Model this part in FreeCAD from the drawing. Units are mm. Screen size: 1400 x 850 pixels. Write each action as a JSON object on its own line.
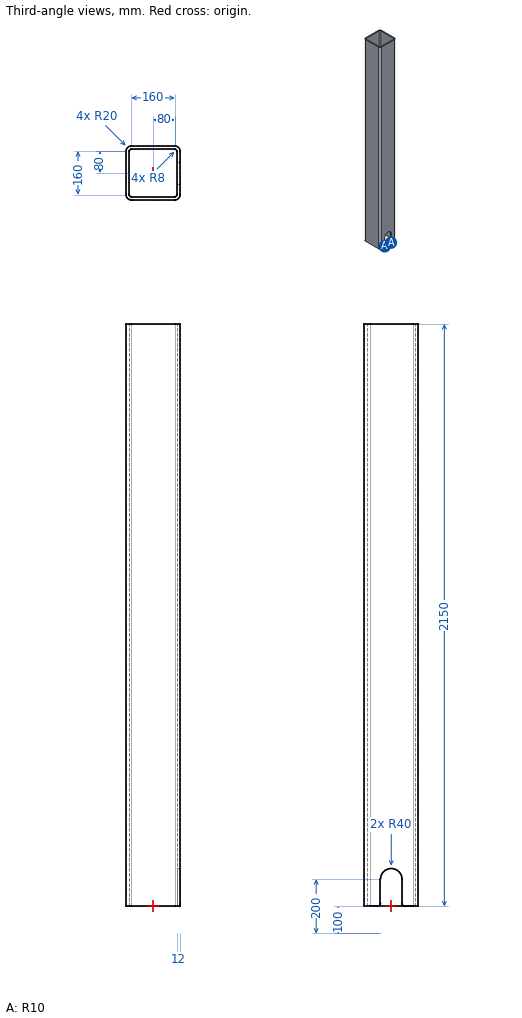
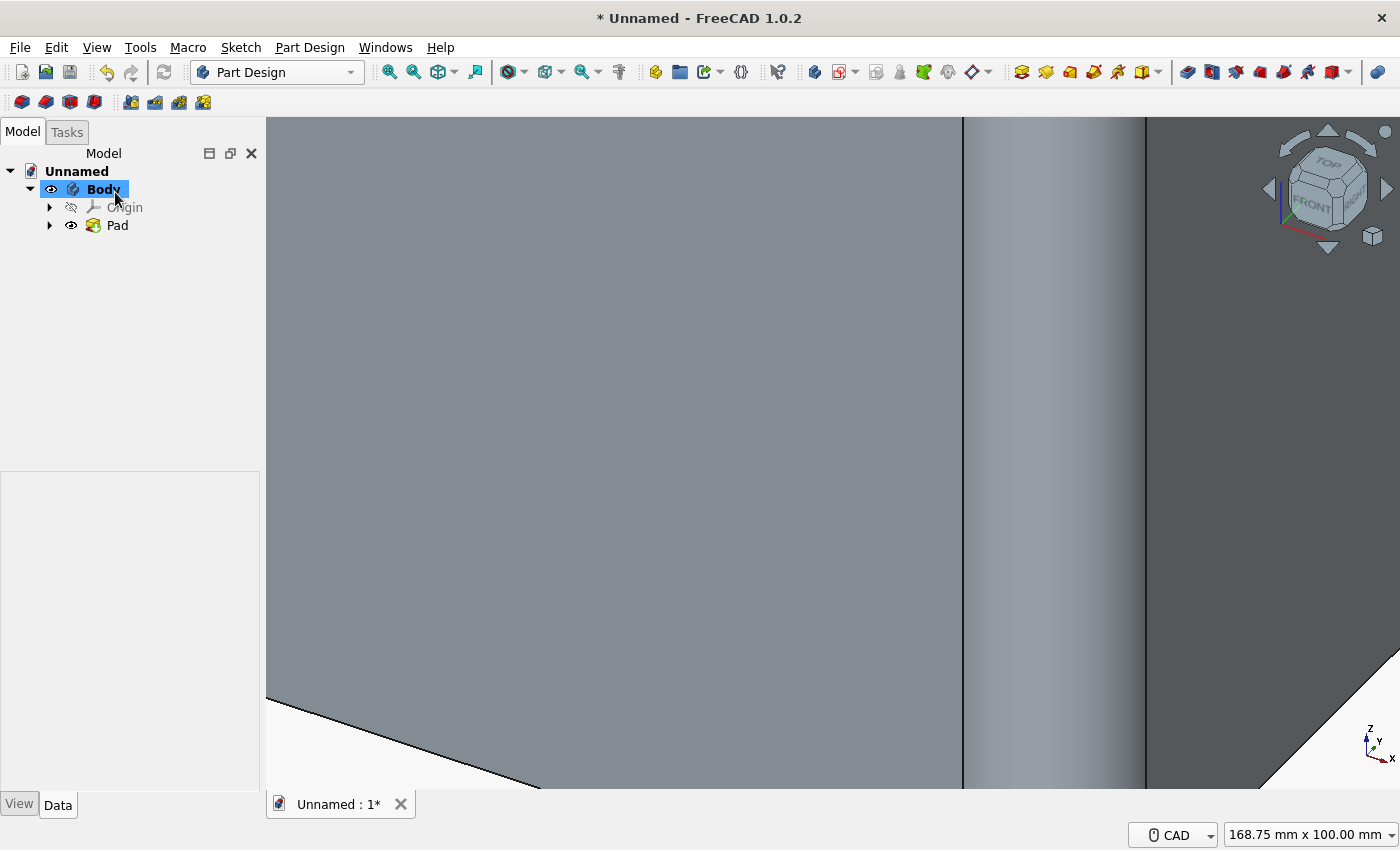
{"action": "left_click", "coordinate": [390, 72]}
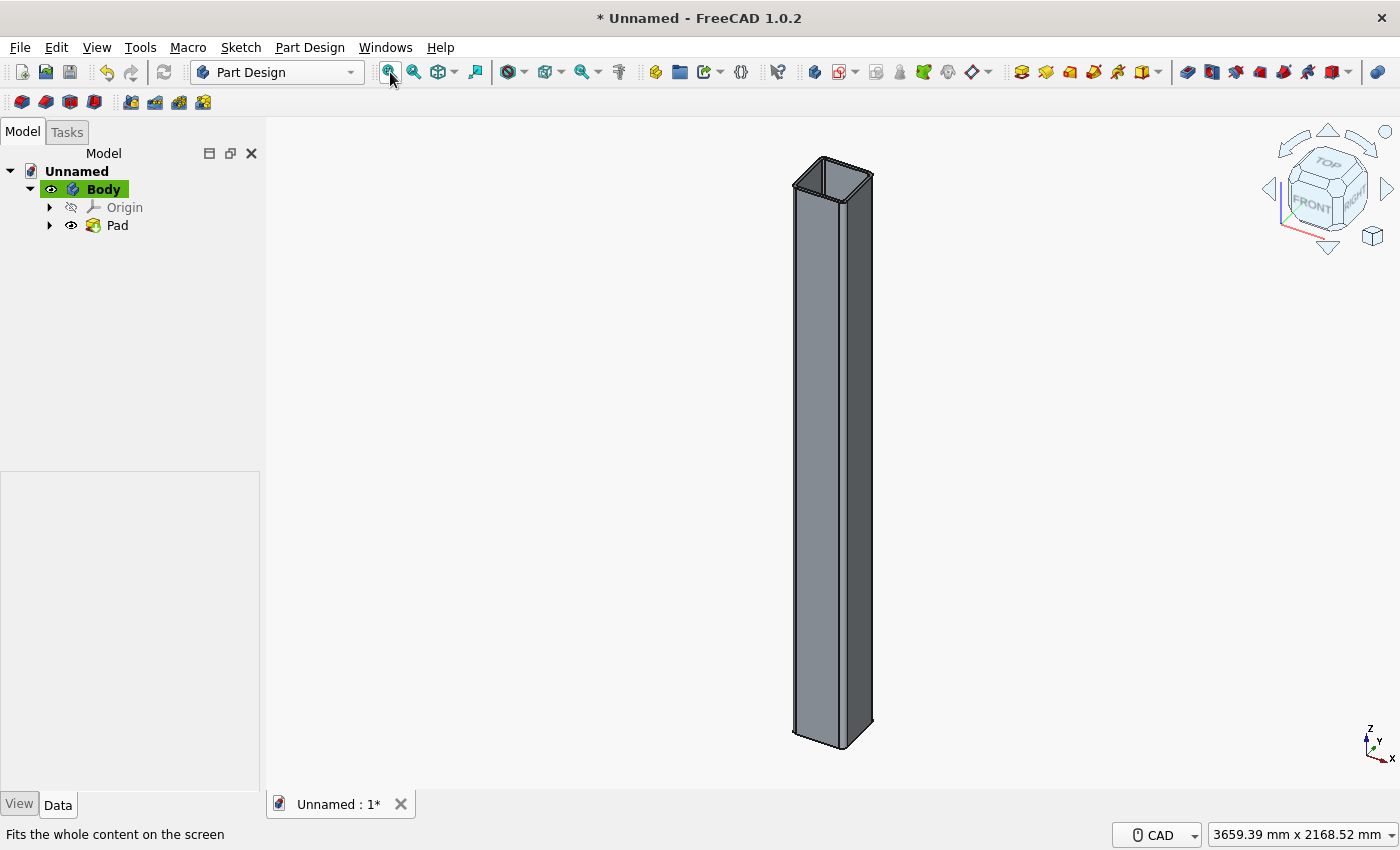
{"action": "left_click", "coordinate": [860, 227]}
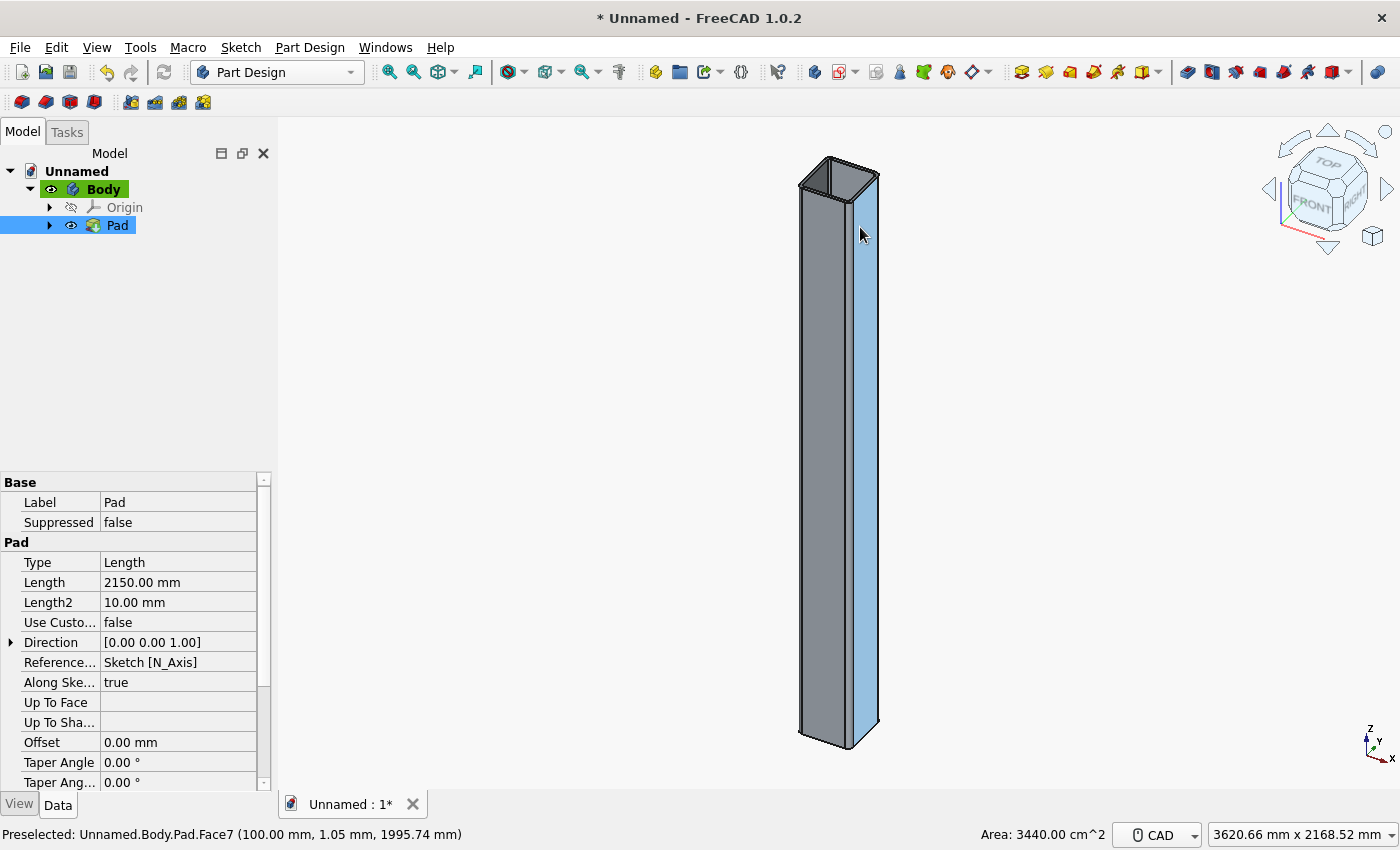
{"action": "left_click", "coordinate": [840, 72]}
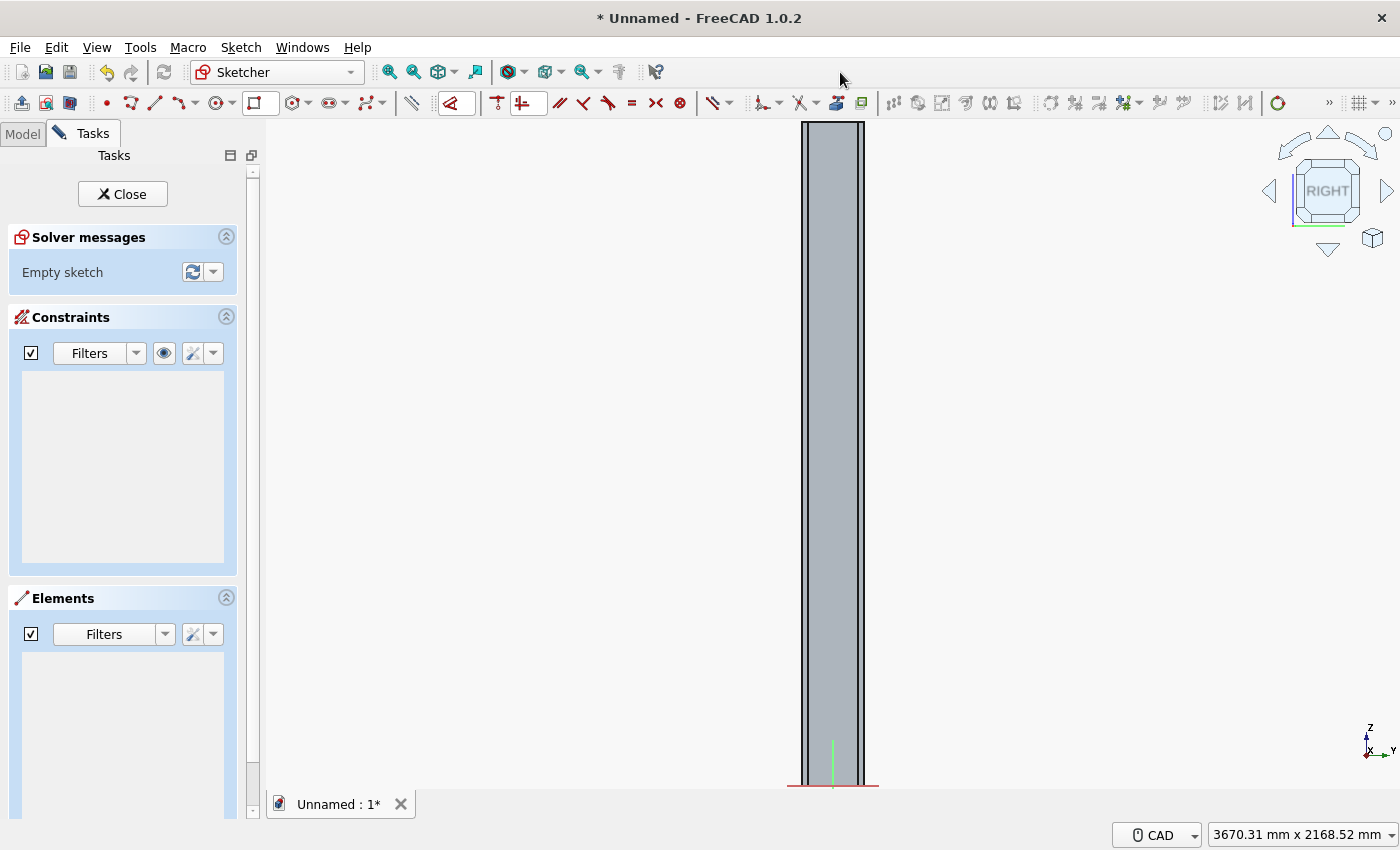
{"action": "scroll", "coordinate": [764, 454], "scroll_direction": "down", "scroll_amount": 5}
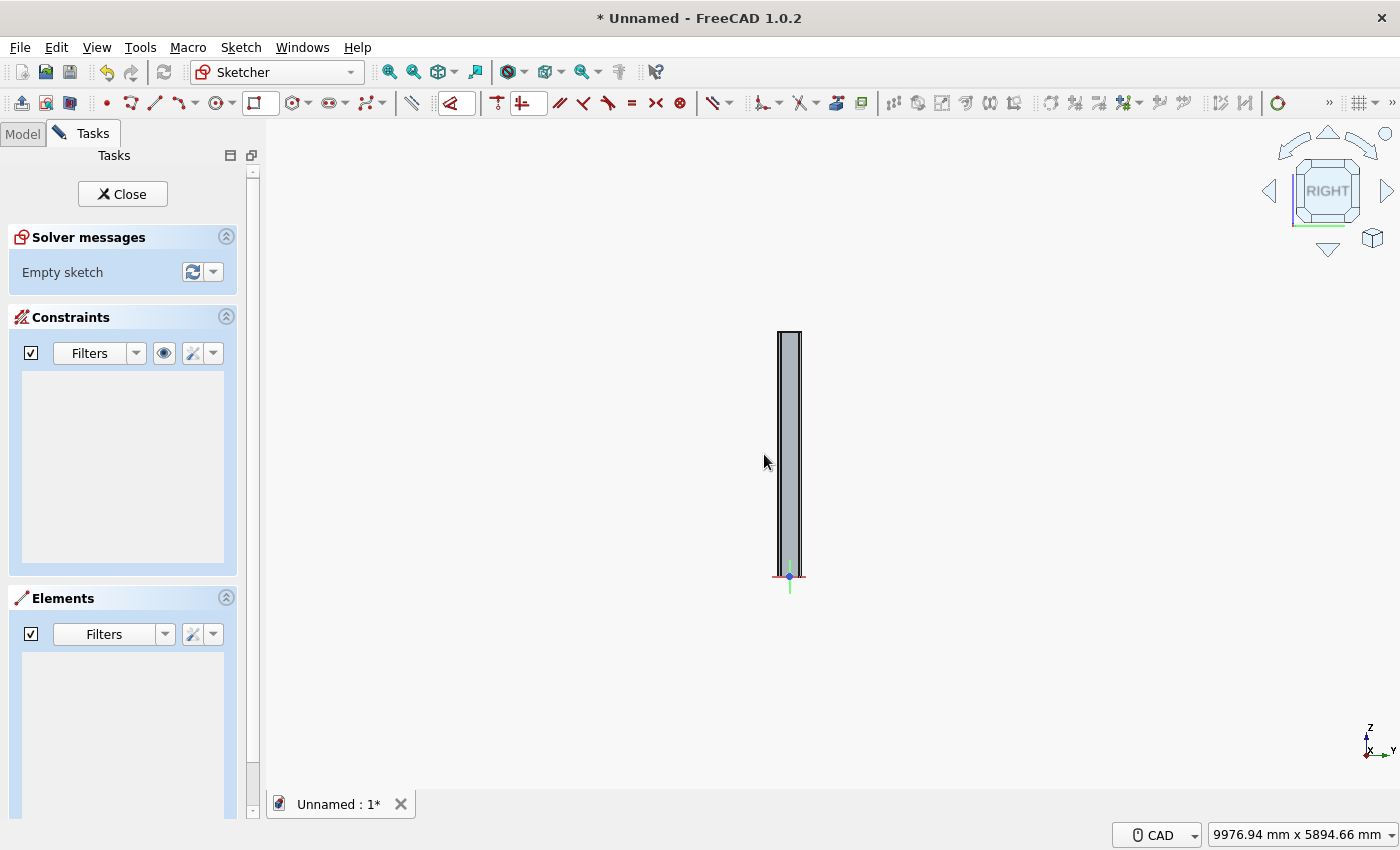
{"action": "scroll", "coordinate": [792, 586], "scroll_direction": "up", "scroll_amount": 13}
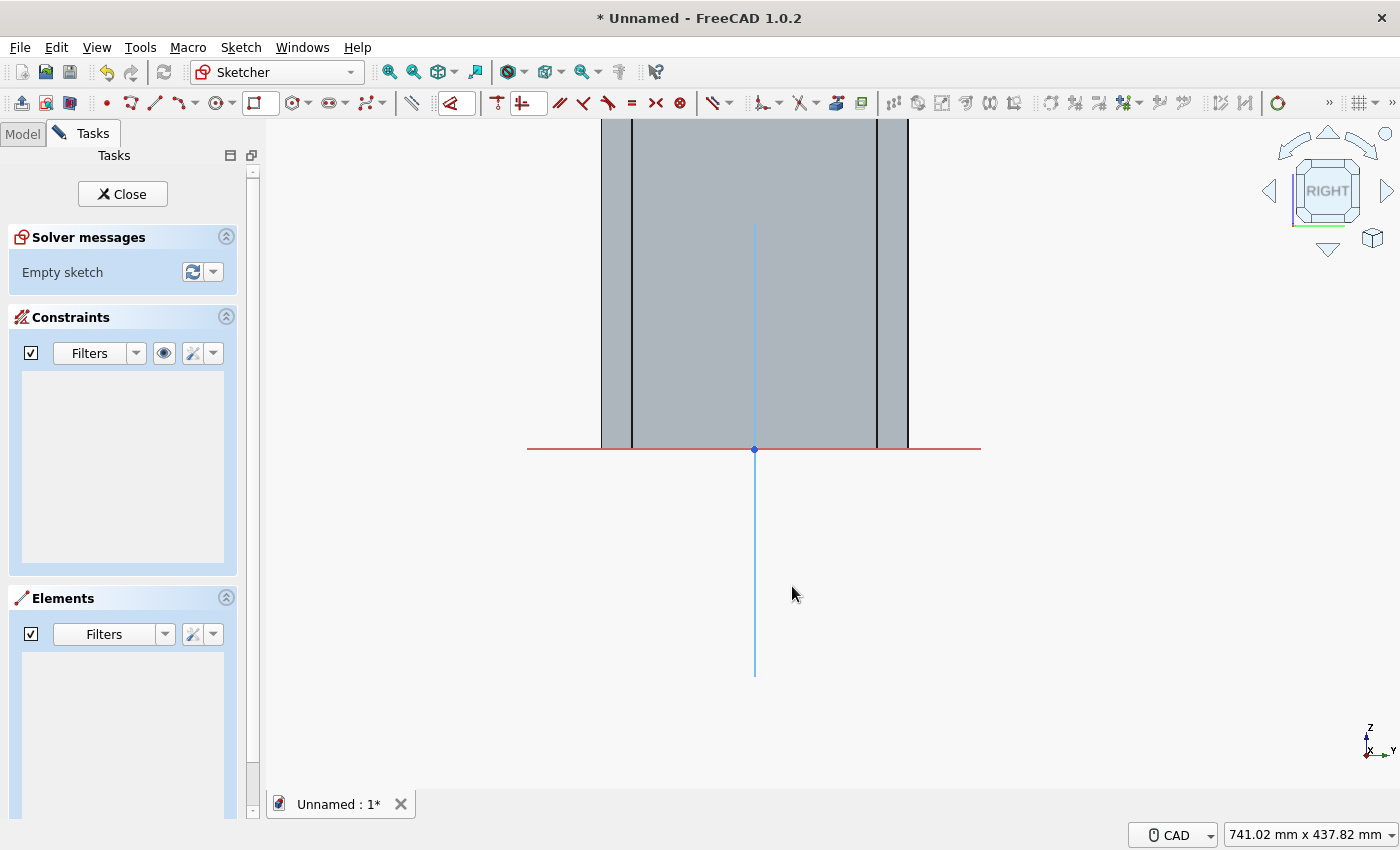
{"action": "left_click", "coordinate": [330, 104]}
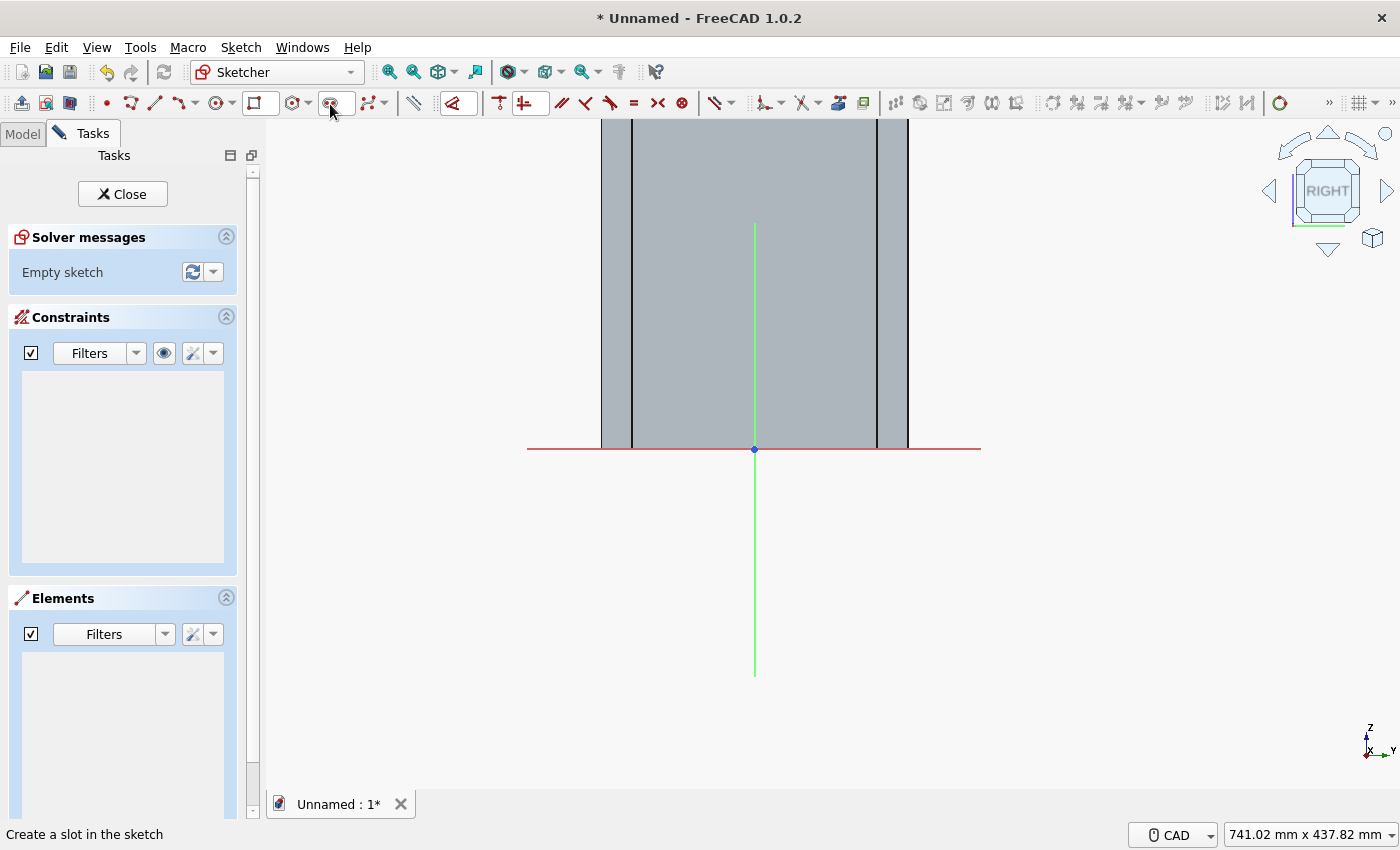
{"action": "left_click", "coordinate": [755, 602]}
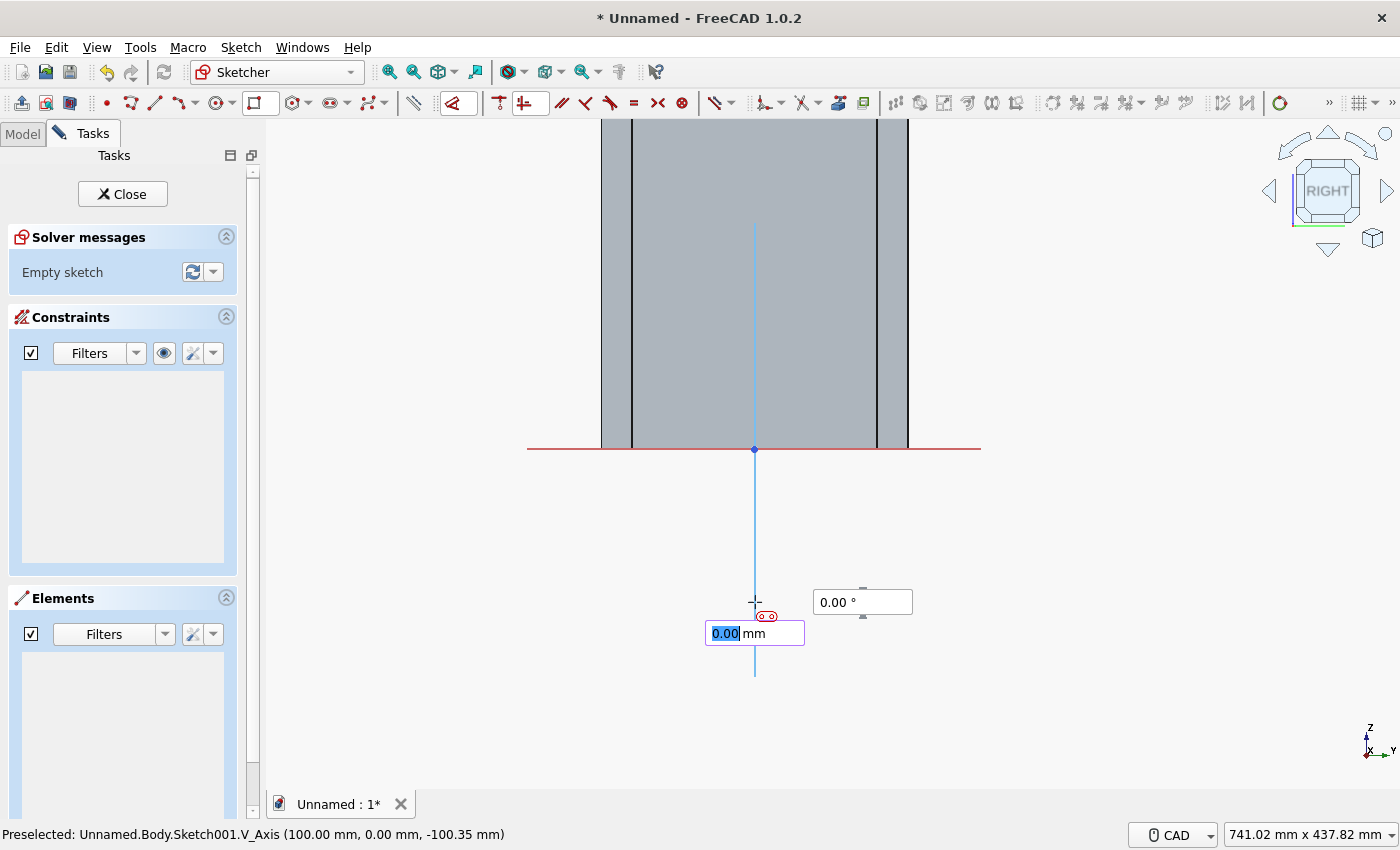
{"action": "left_click", "coordinate": [764, 296]}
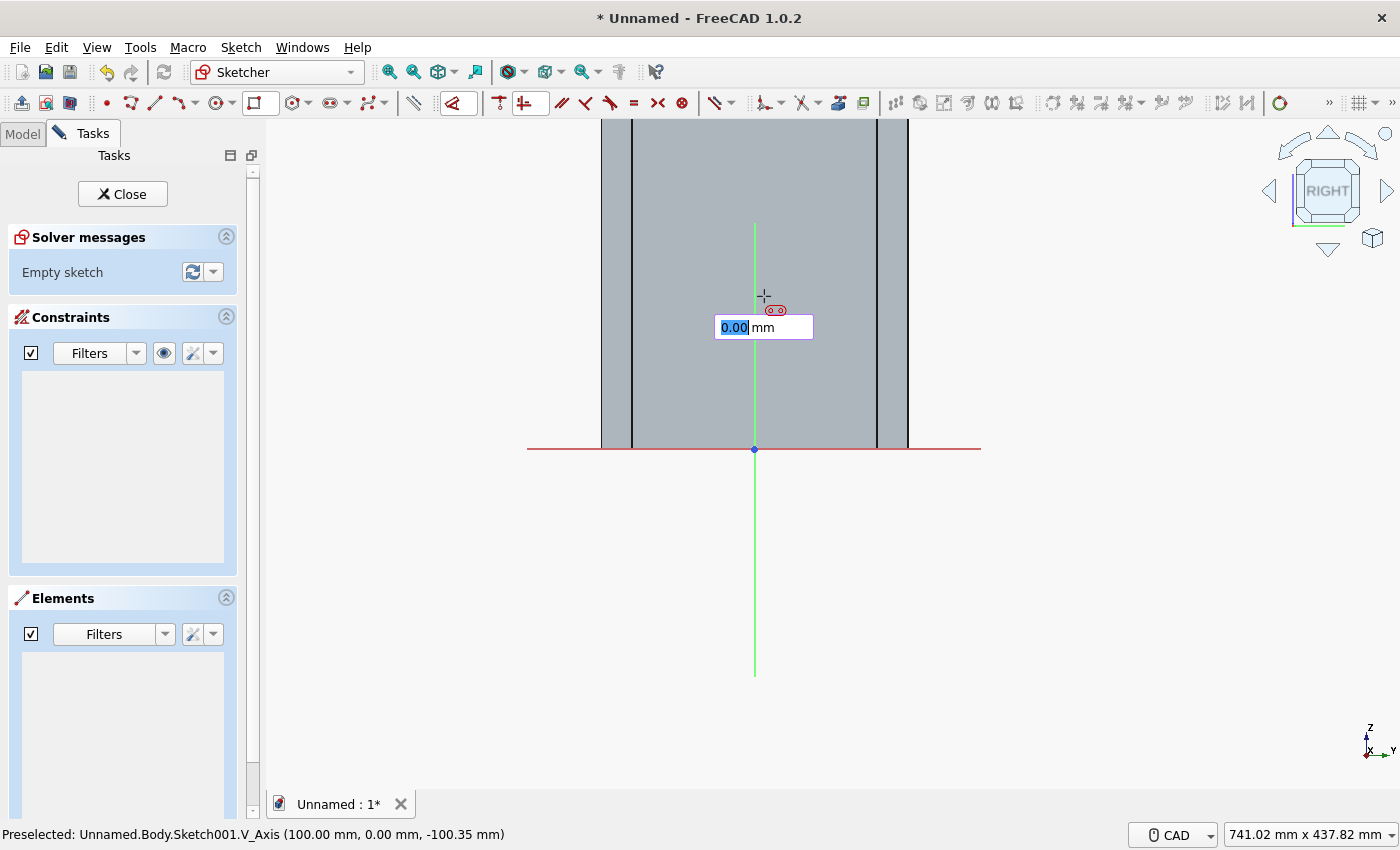
{"action": "left_click", "coordinate": [816, 495]}
{"action": "key", "text": "Escape"}